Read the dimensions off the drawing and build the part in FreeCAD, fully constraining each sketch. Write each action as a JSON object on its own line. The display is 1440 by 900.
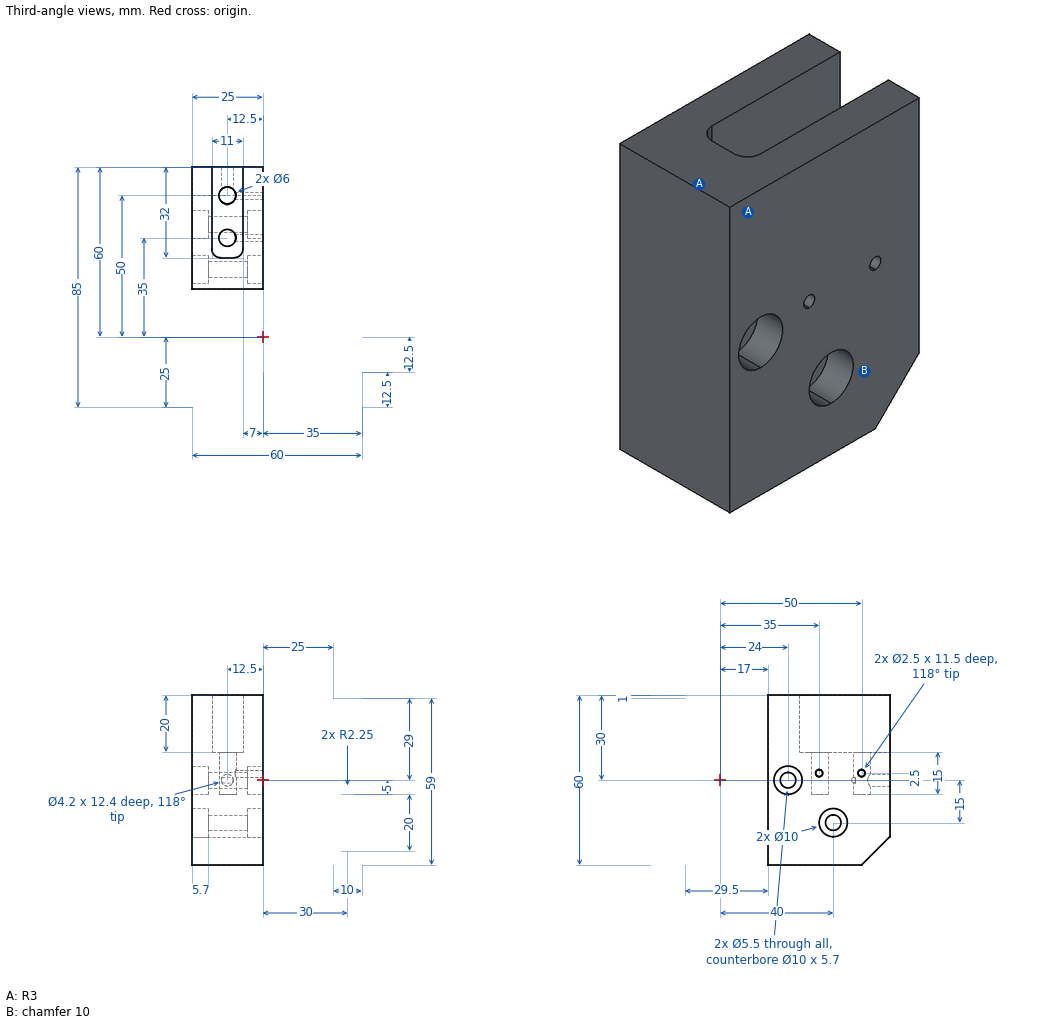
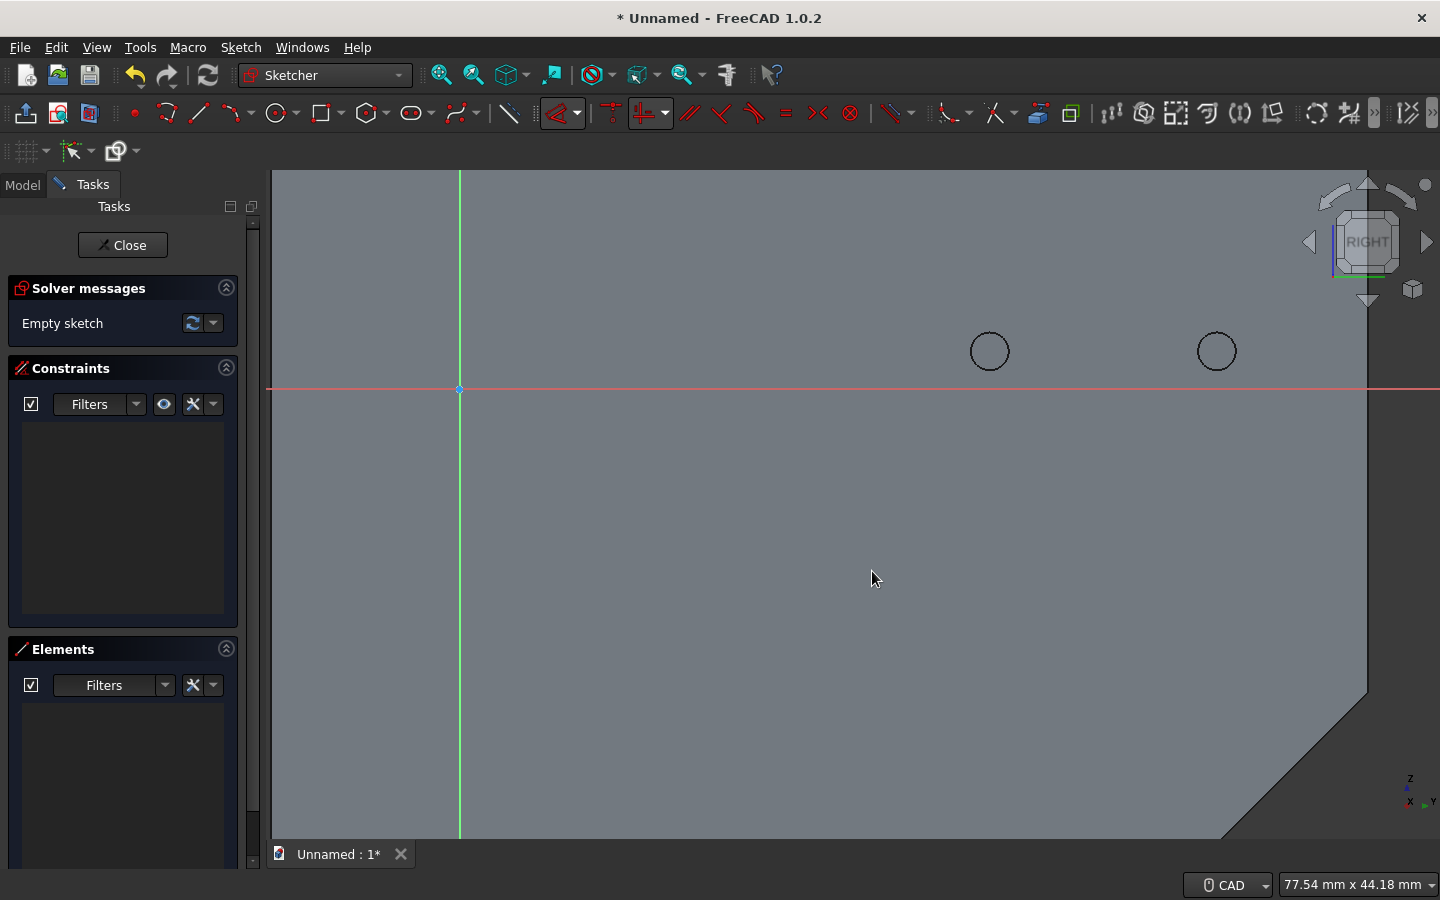
{"action": "left_click", "coordinate": [276, 114]}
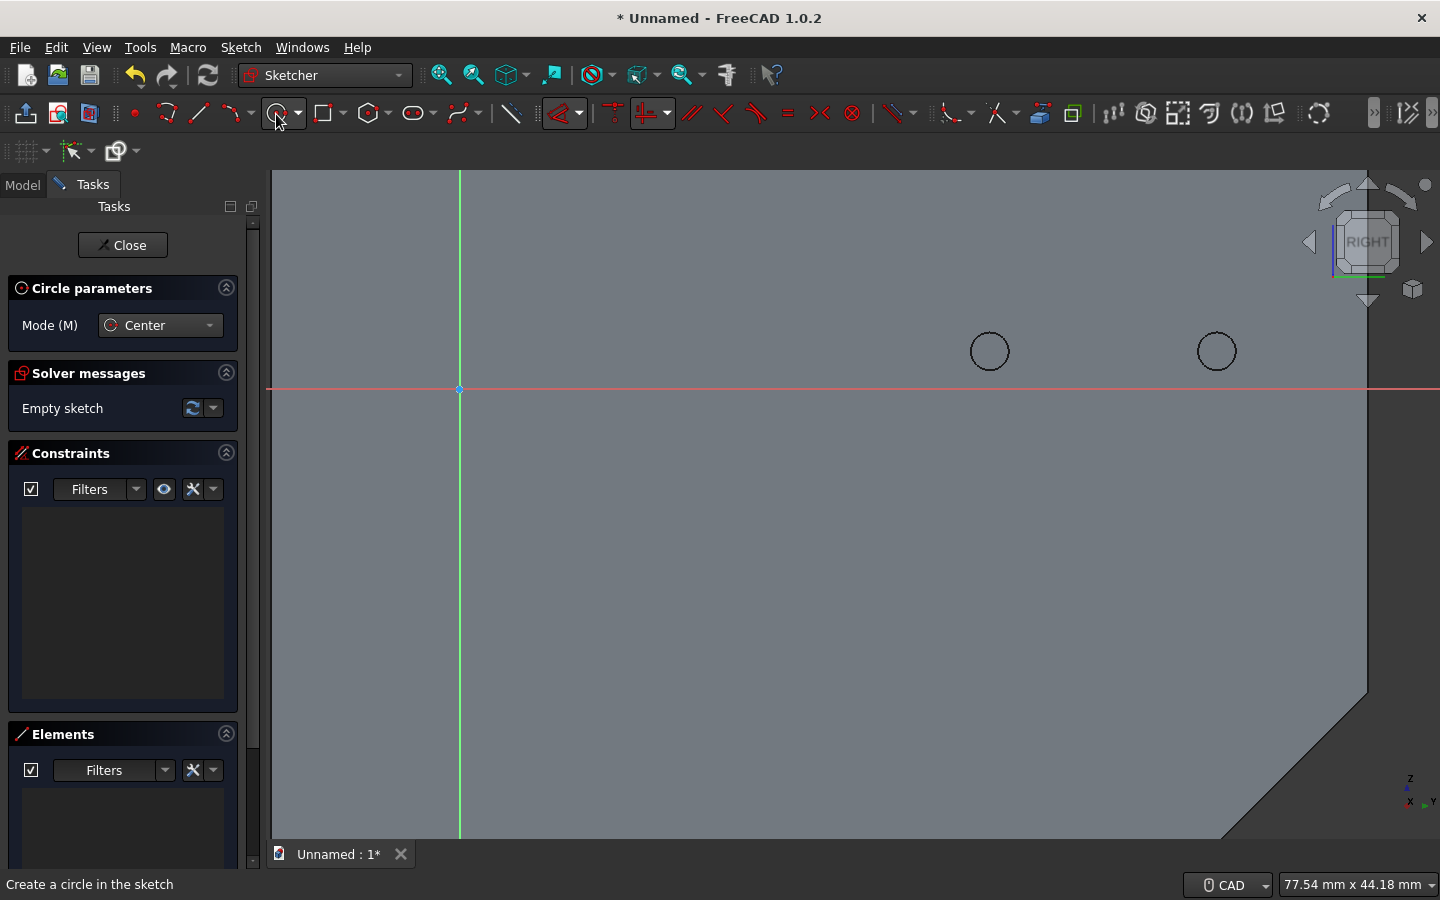
{"action": "left_click", "coordinate": [823, 389]}
{"action": "mouse_move", "coordinate": [853, 360]}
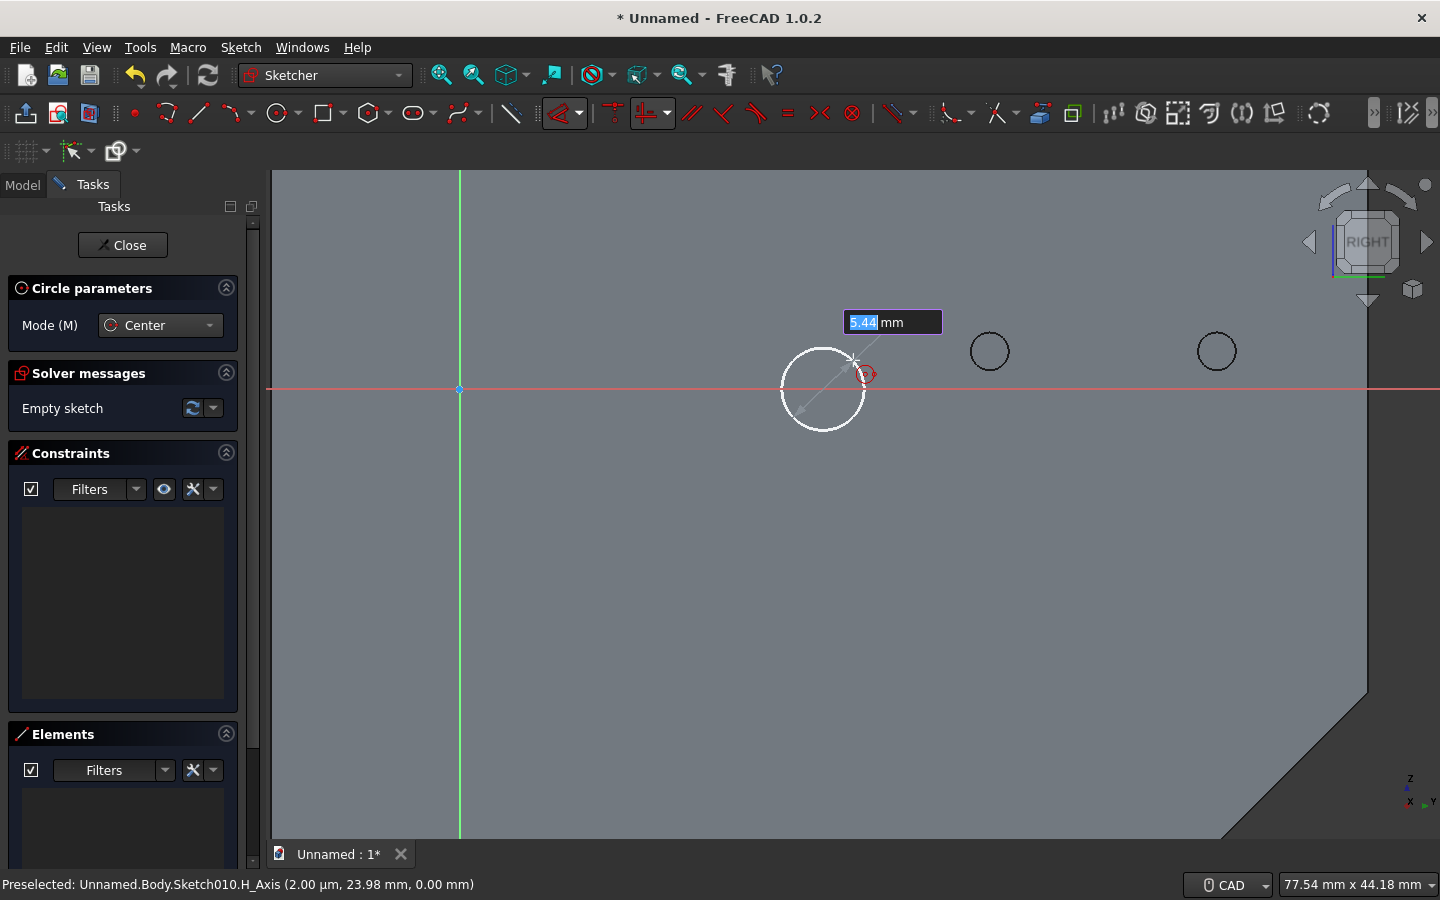
{"action": "type", "text": "5.5"}
{"action": "key", "text": "Return"}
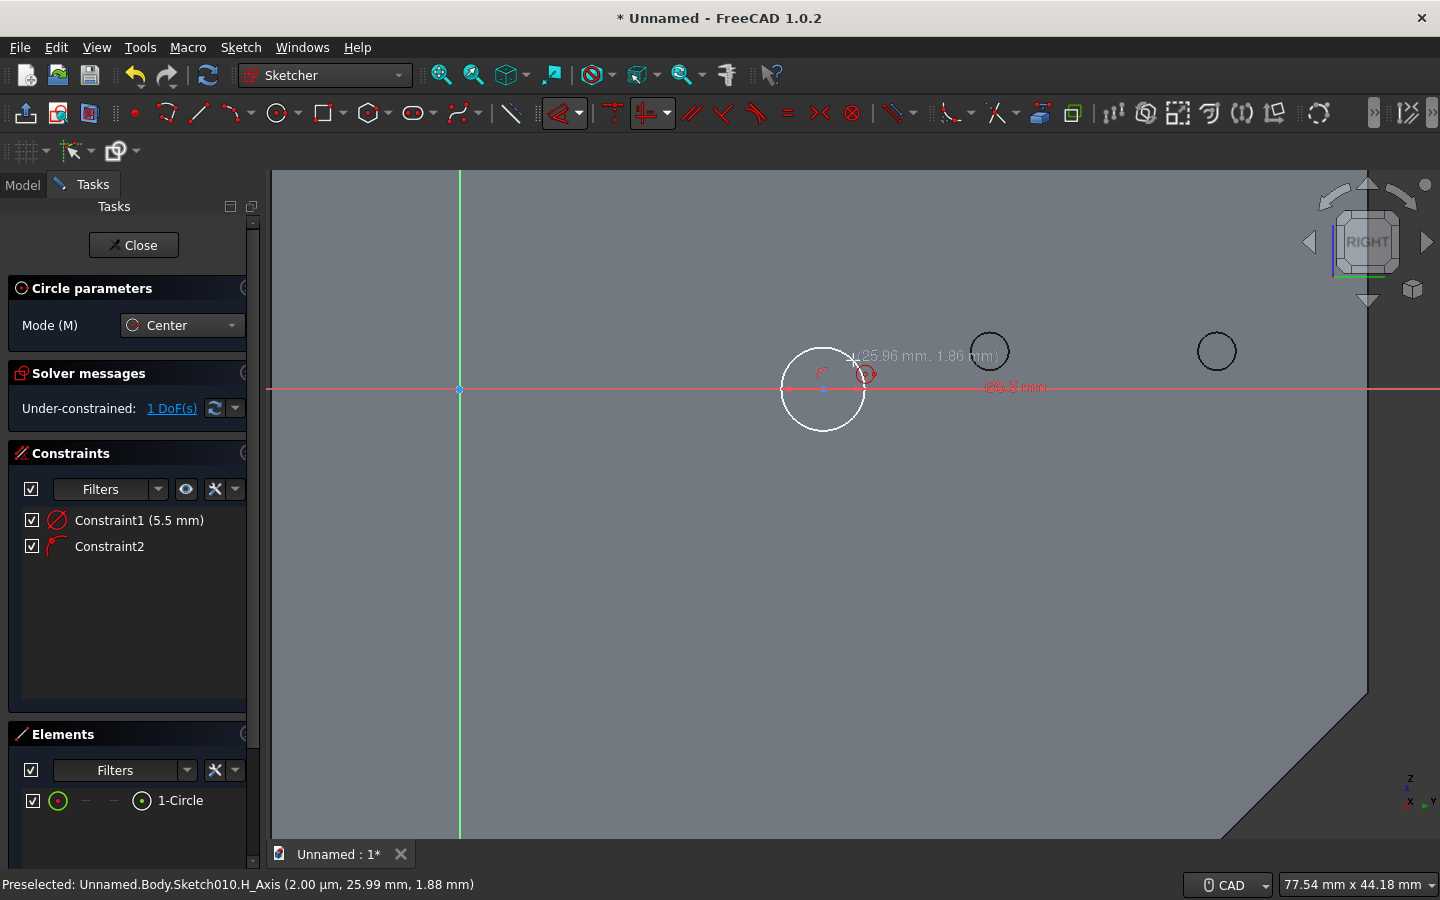
{"action": "left_click", "coordinate": [1066, 616]}
{"action": "mouse_move", "coordinate": [1095, 587]}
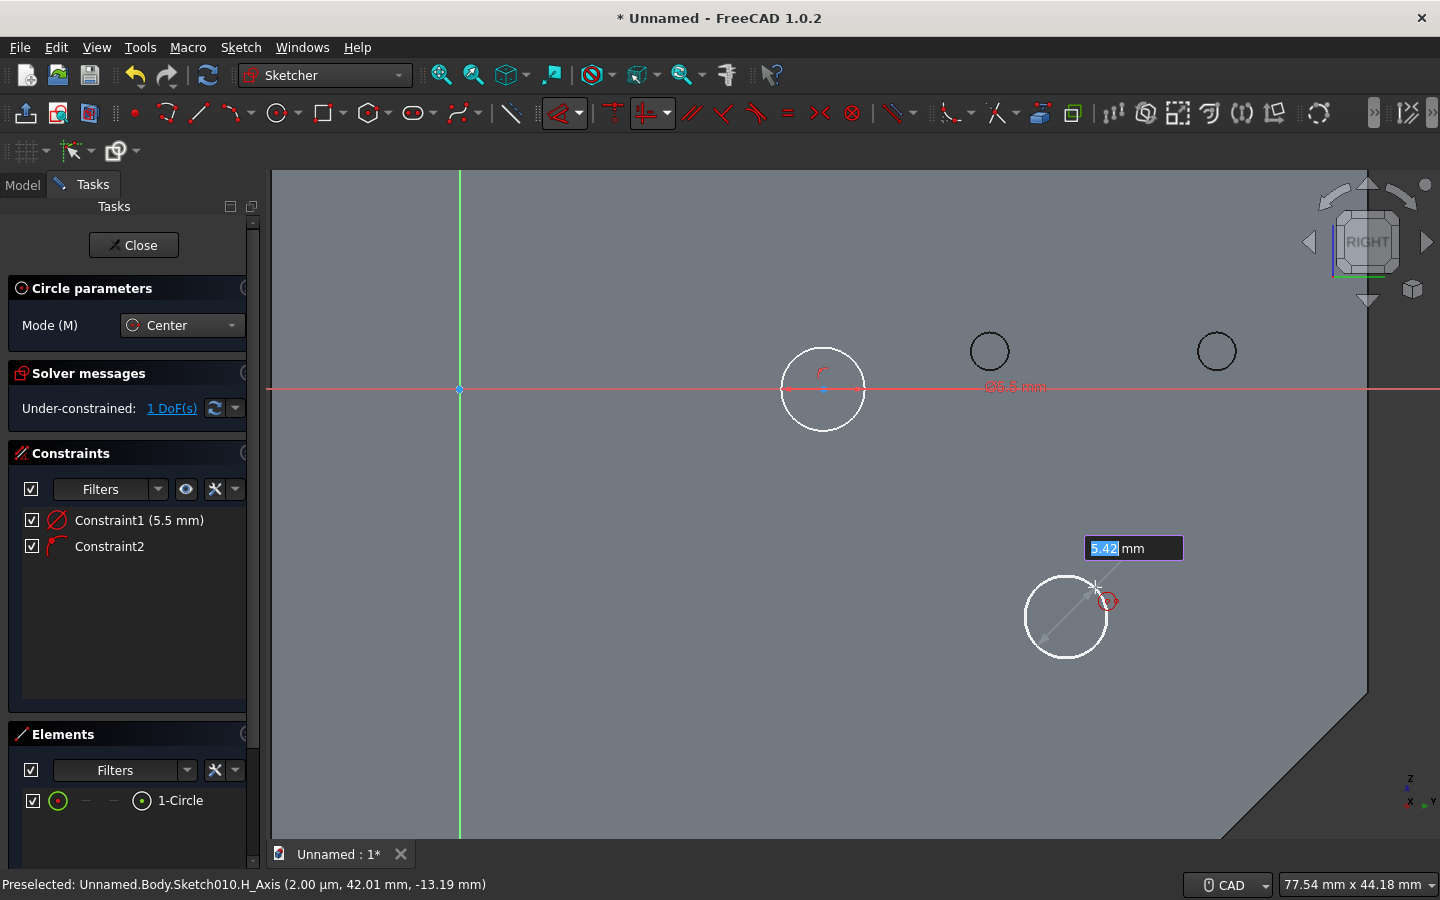
{"action": "type", "text": "5.5"}
{"action": "key", "text": "Return"}
{"action": "key", "text": "Escape"}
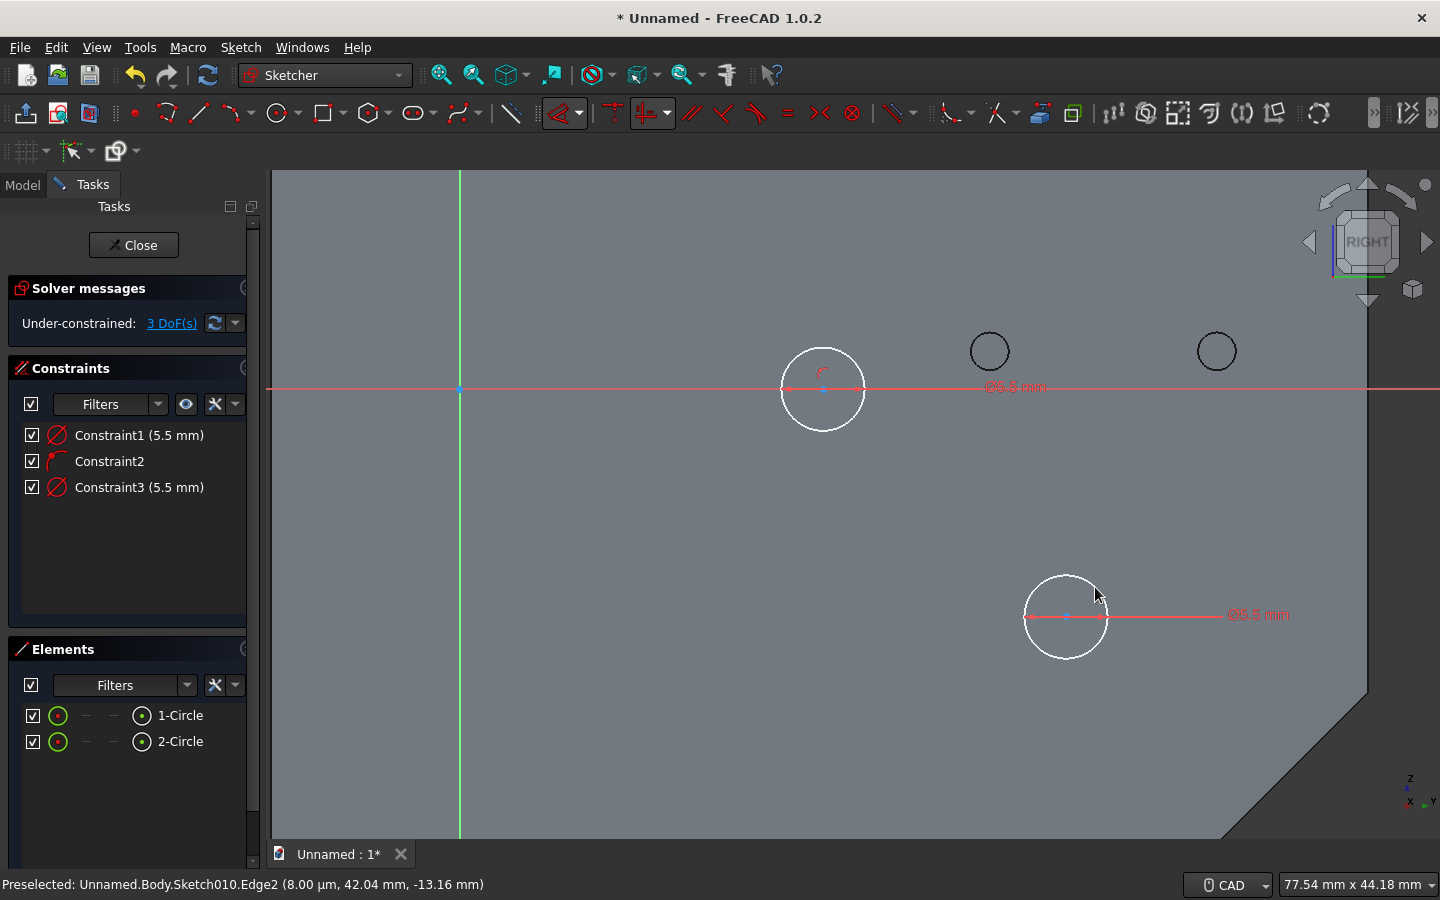
{"action": "left_click", "coordinate": [823, 389]}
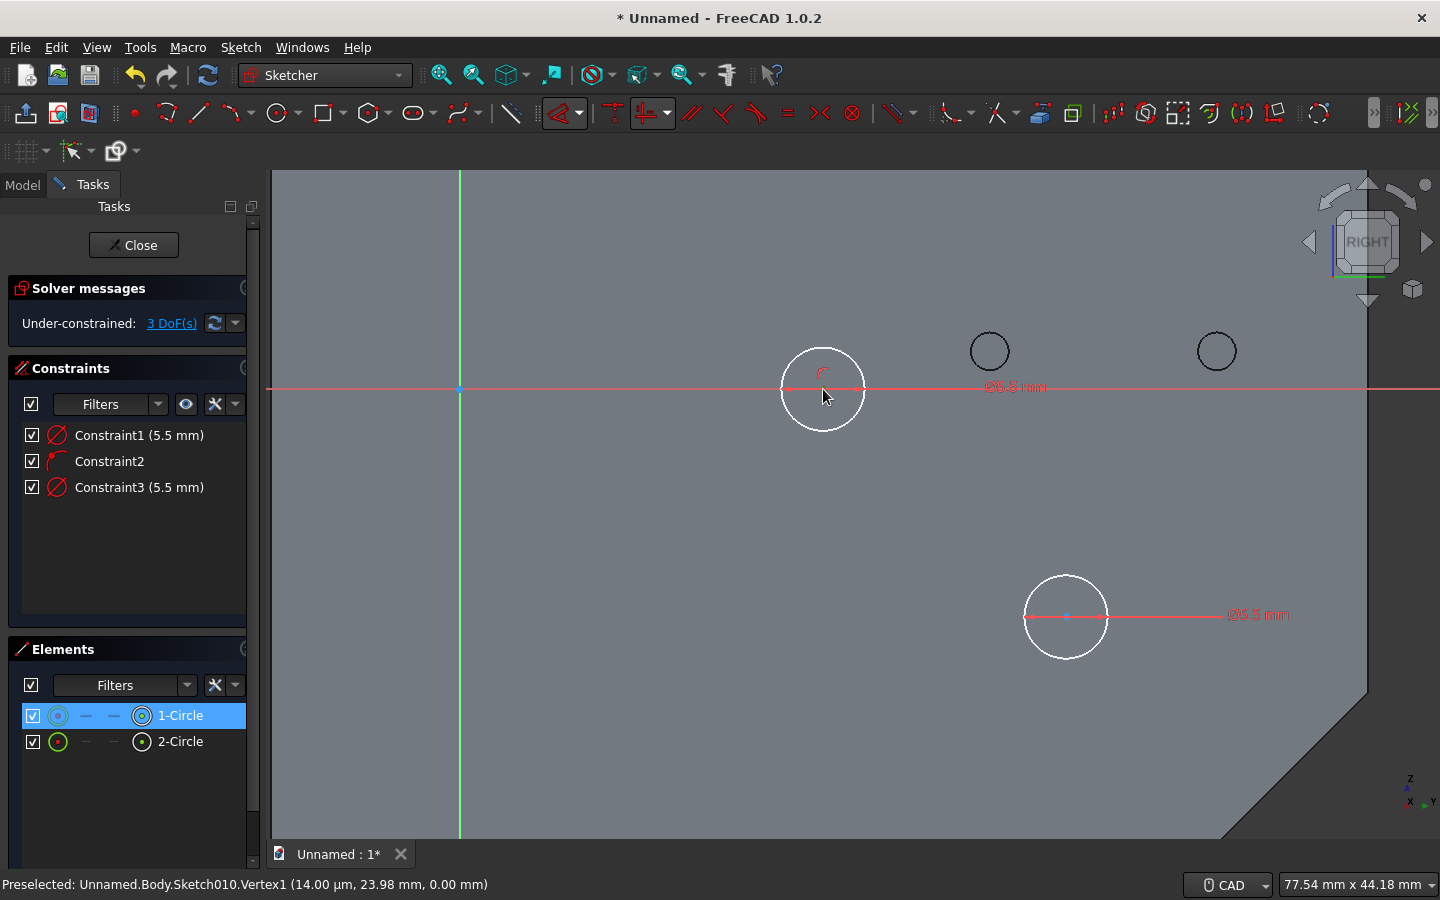
{"action": "left_click", "coordinate": [582, 114]}